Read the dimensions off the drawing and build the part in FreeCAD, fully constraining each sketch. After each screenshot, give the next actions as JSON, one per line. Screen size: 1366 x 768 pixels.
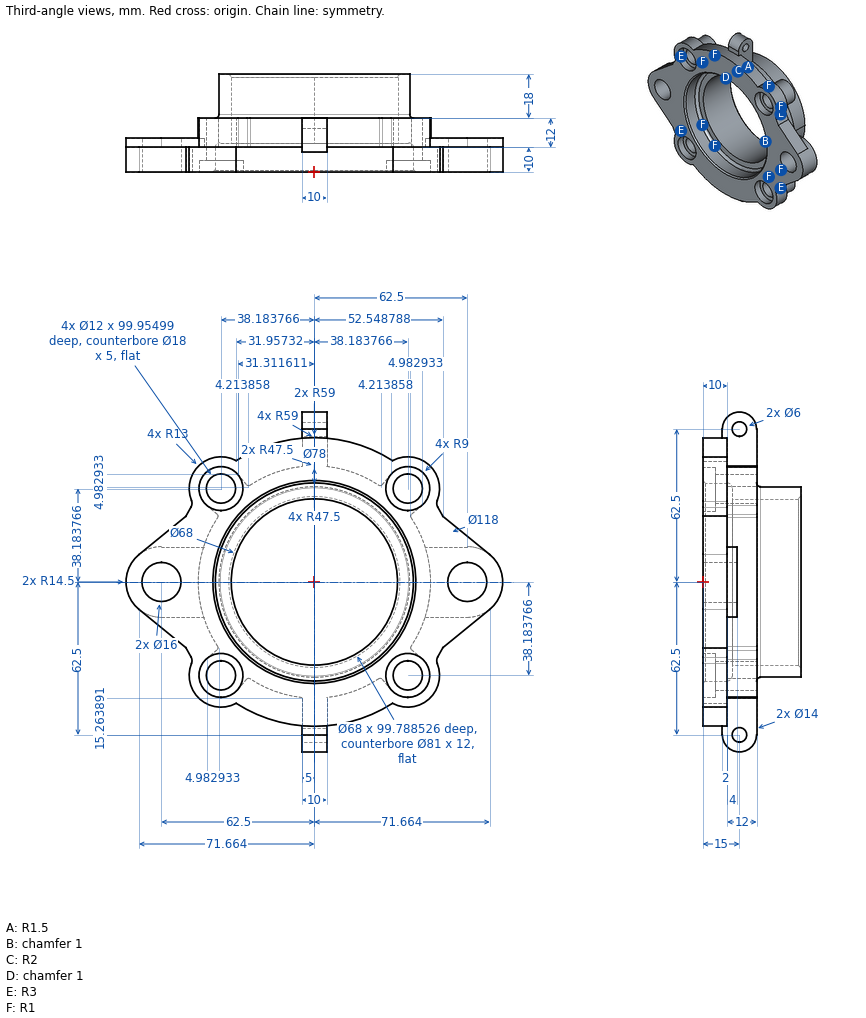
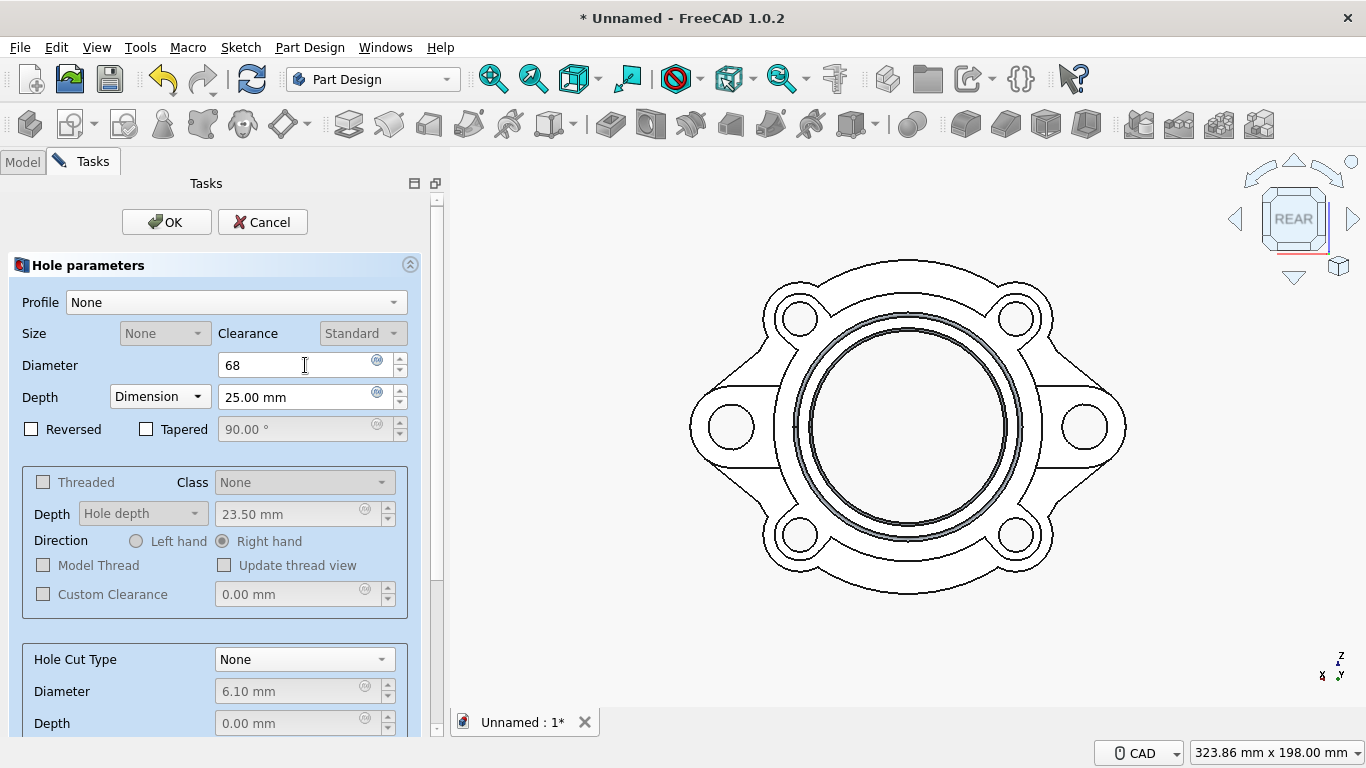
{"action": "triple_click", "coordinate": [305, 397]}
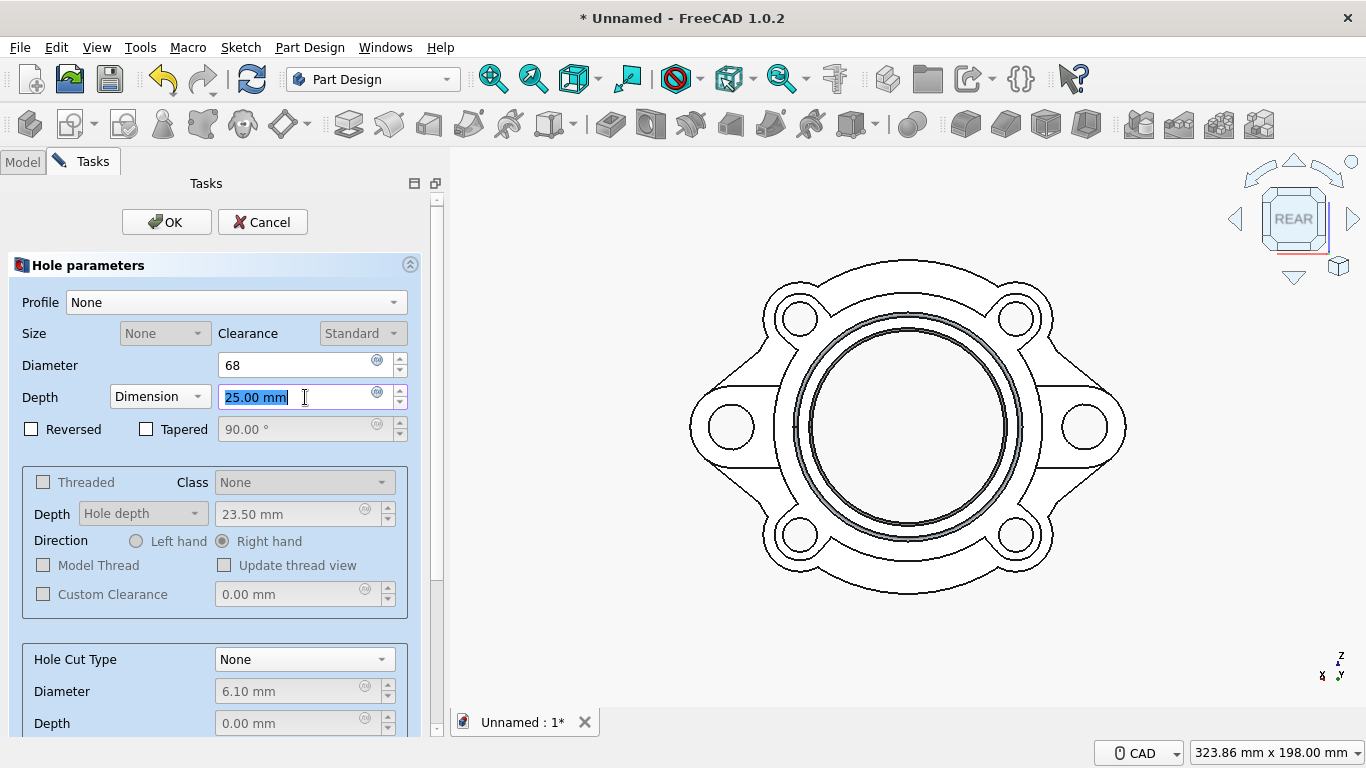
{"action": "type", "text": "99.788526"}
{"action": "key", "text": "Tab"}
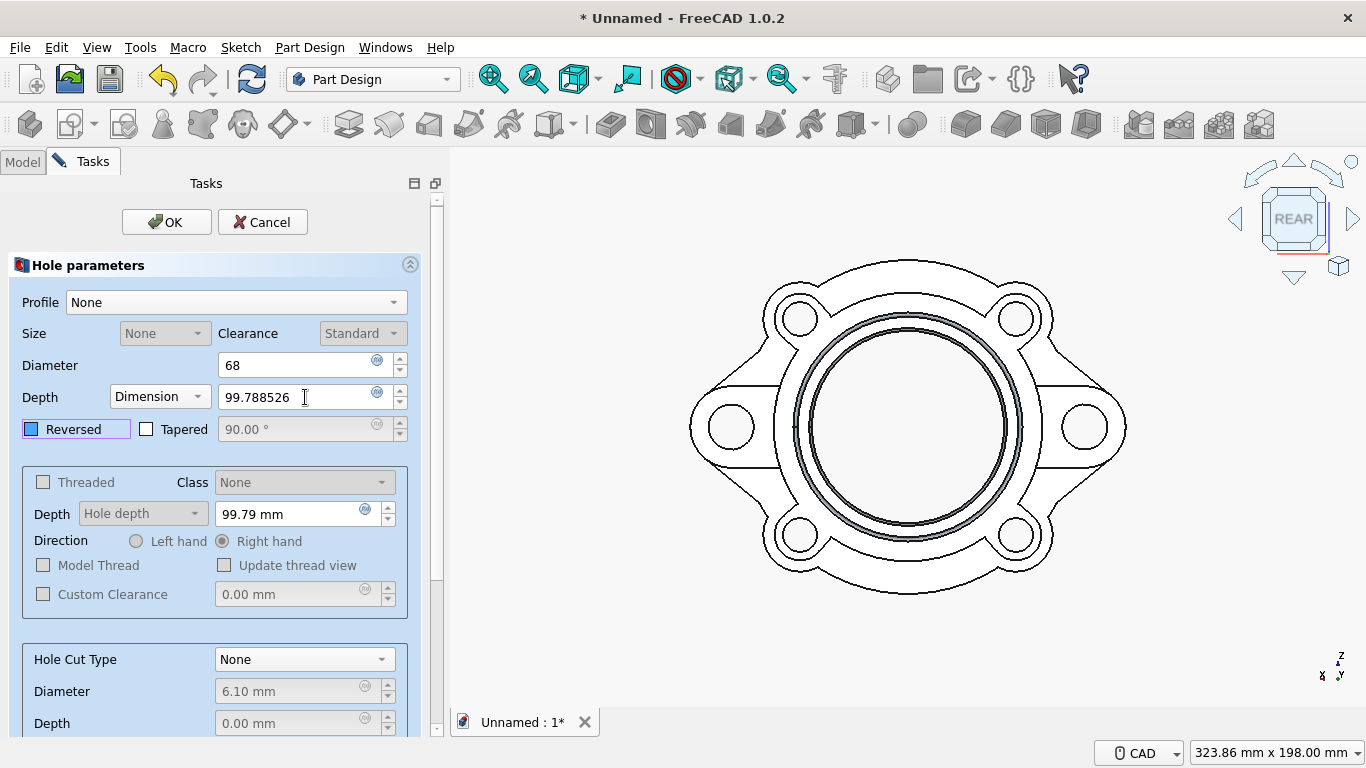
{"action": "left_click", "coordinate": [306, 660]}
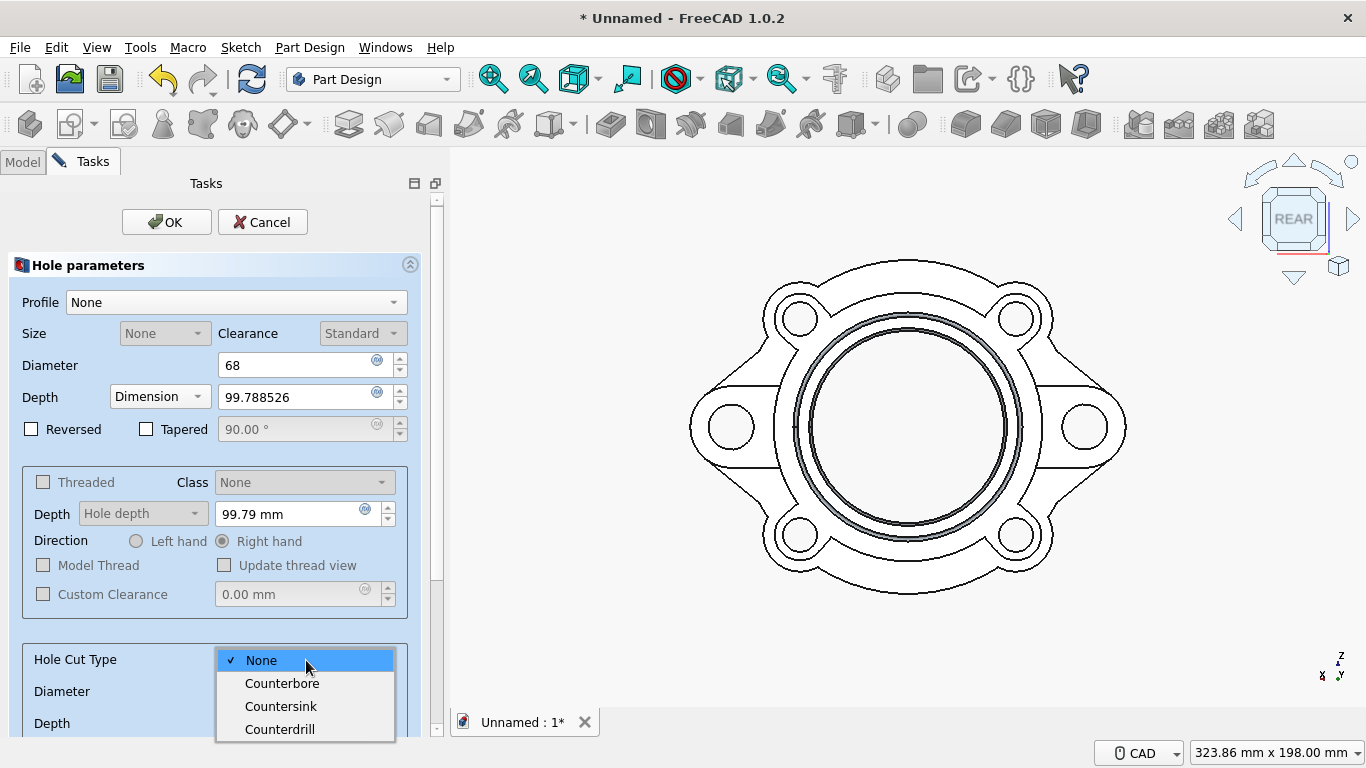
{"action": "left_click", "coordinate": [304, 684]}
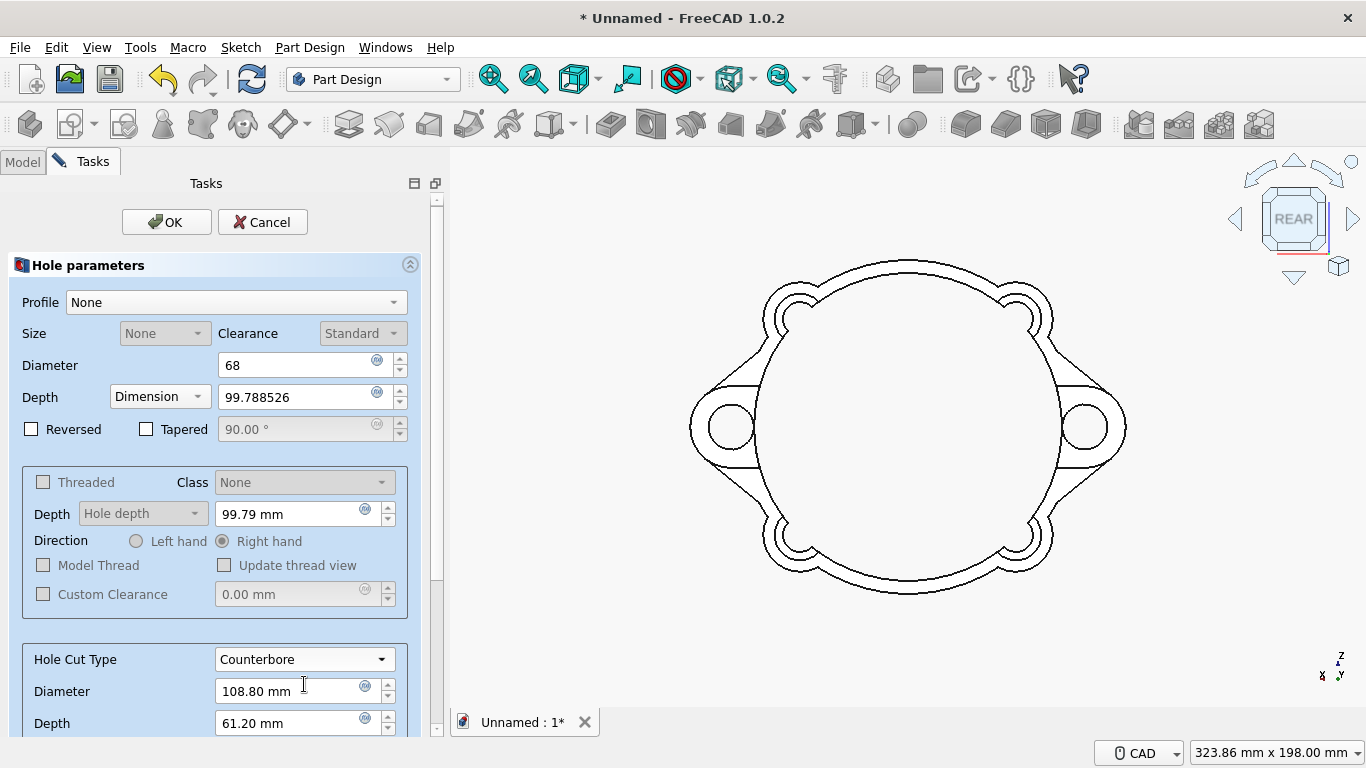
{"action": "triple_click", "coordinate": [298, 691]}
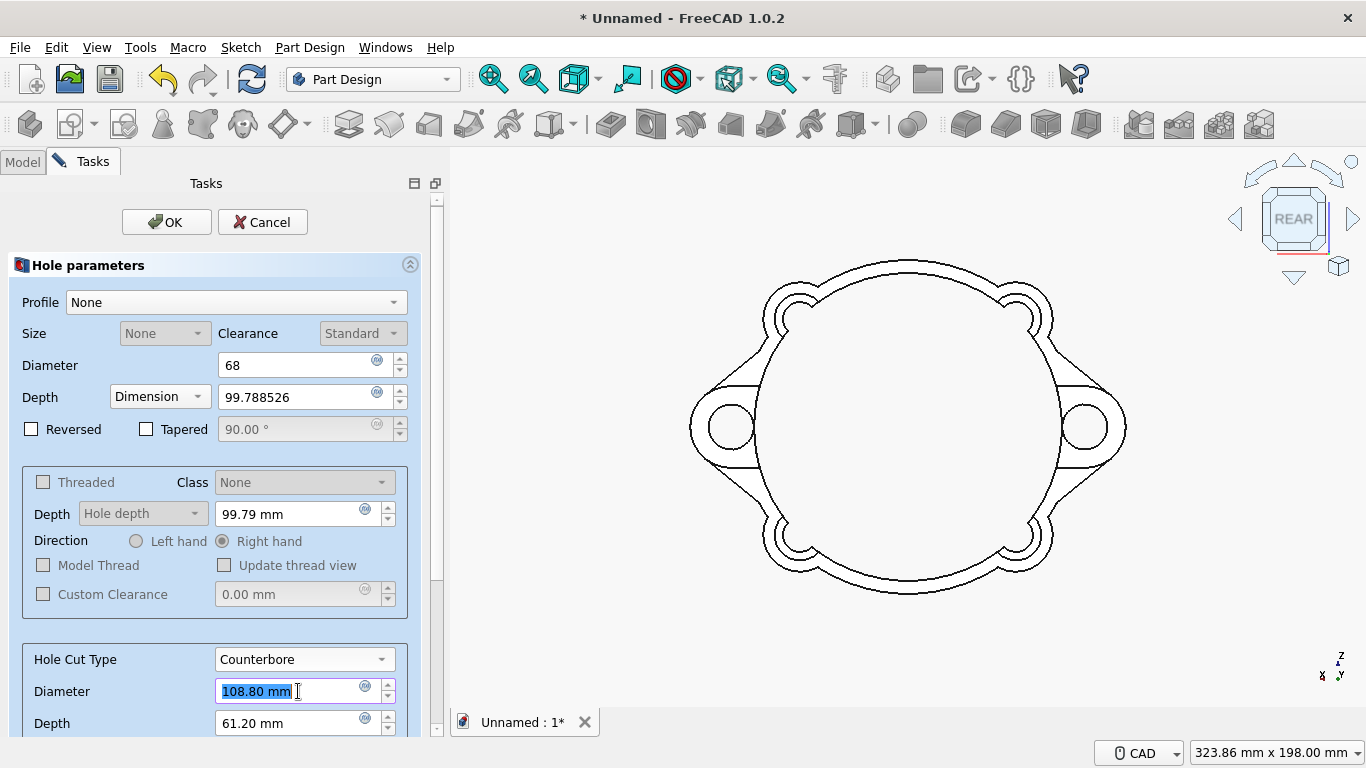
{"action": "type", "text": "81"}
{"action": "key", "text": "Tab"}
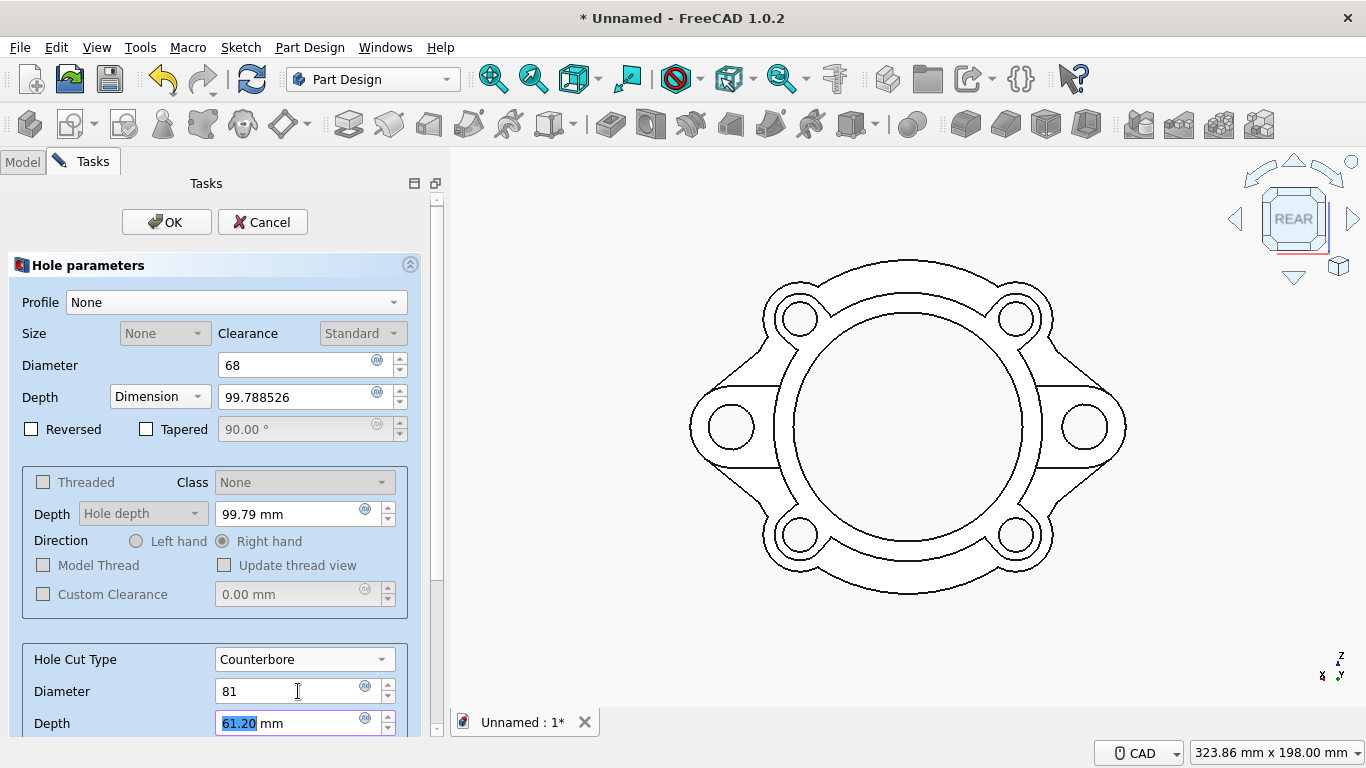
{"action": "type", "text": "12"}
{"action": "key", "text": "Tab"}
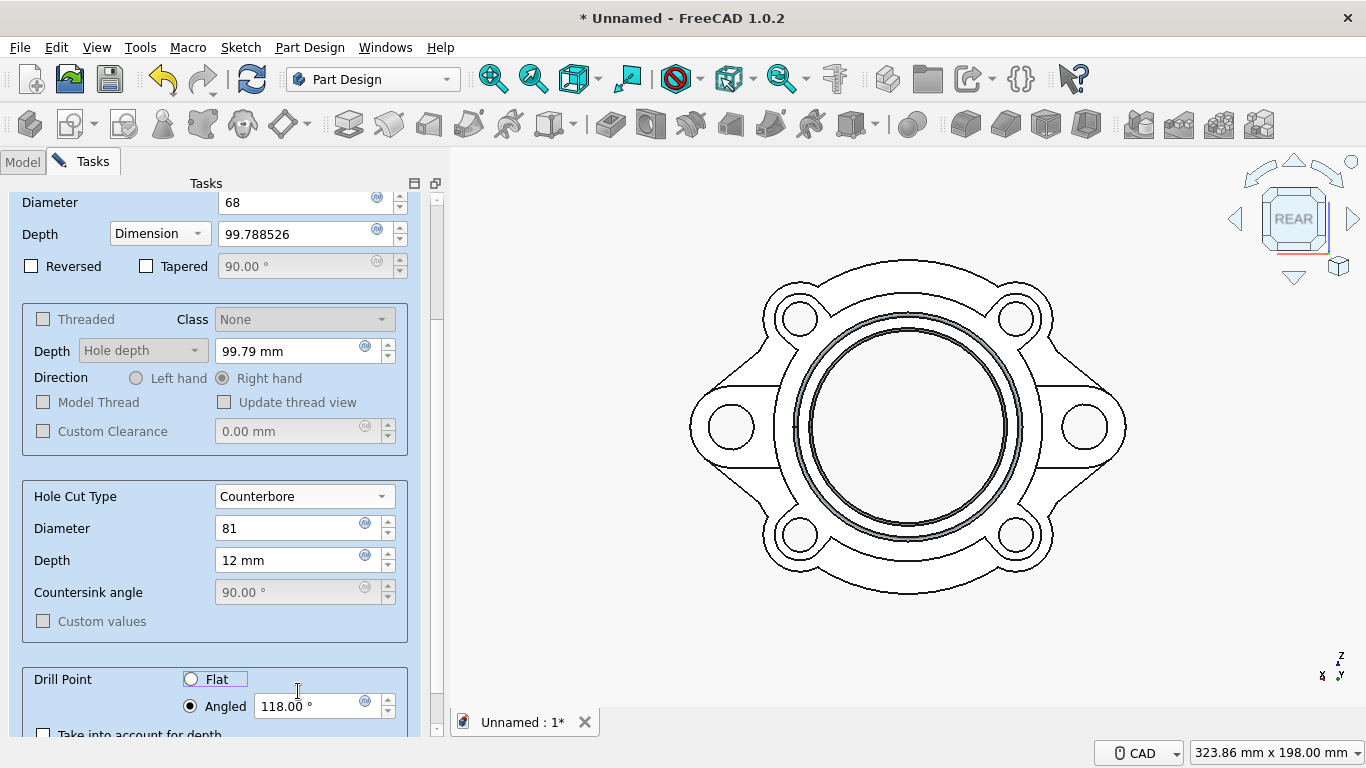
{"action": "left_click", "coordinate": [191, 679]}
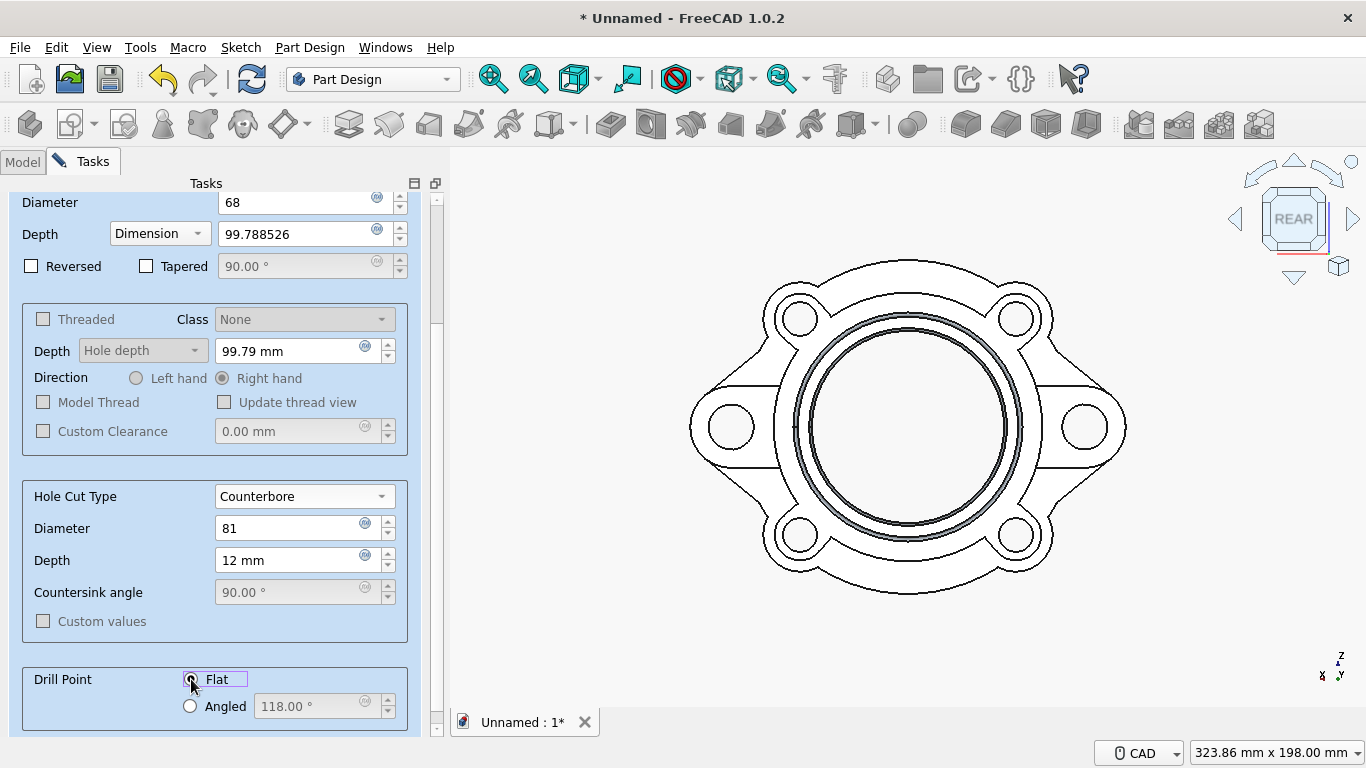
{"action": "scroll", "coordinate": [437, 464], "scroll_direction": "up", "scroll_amount": 4}